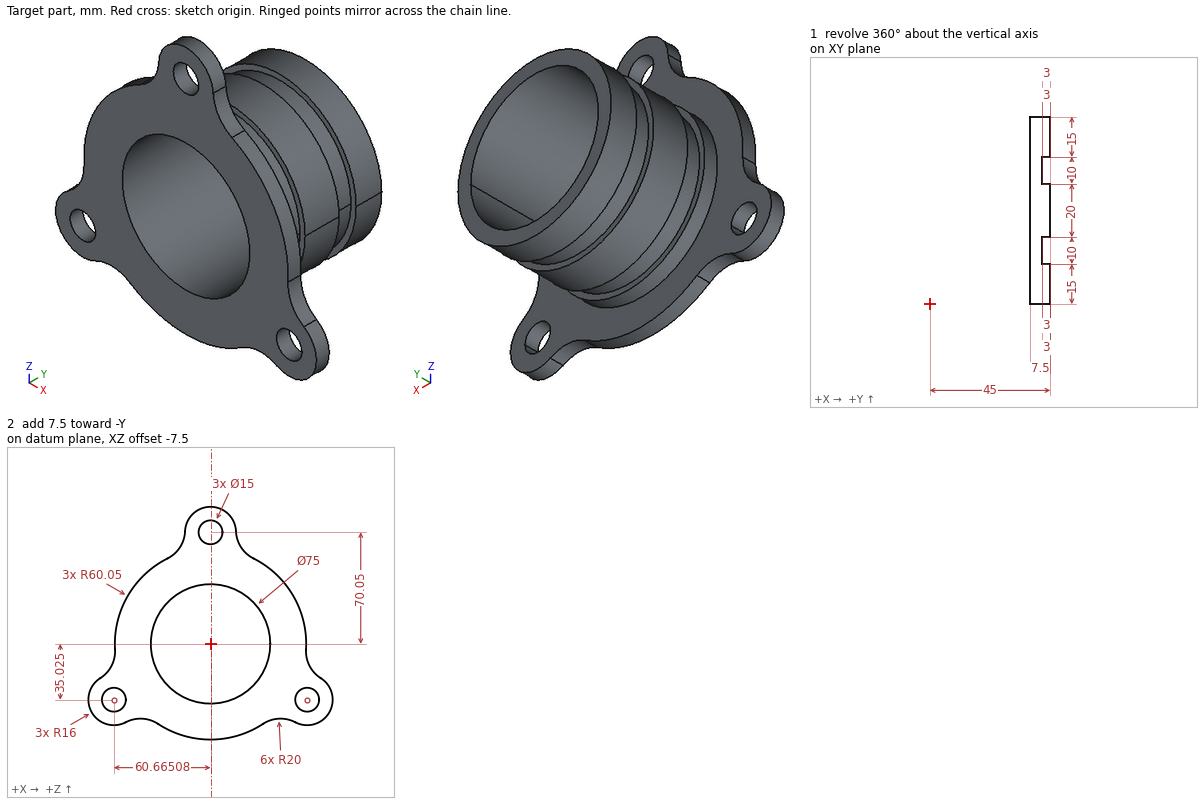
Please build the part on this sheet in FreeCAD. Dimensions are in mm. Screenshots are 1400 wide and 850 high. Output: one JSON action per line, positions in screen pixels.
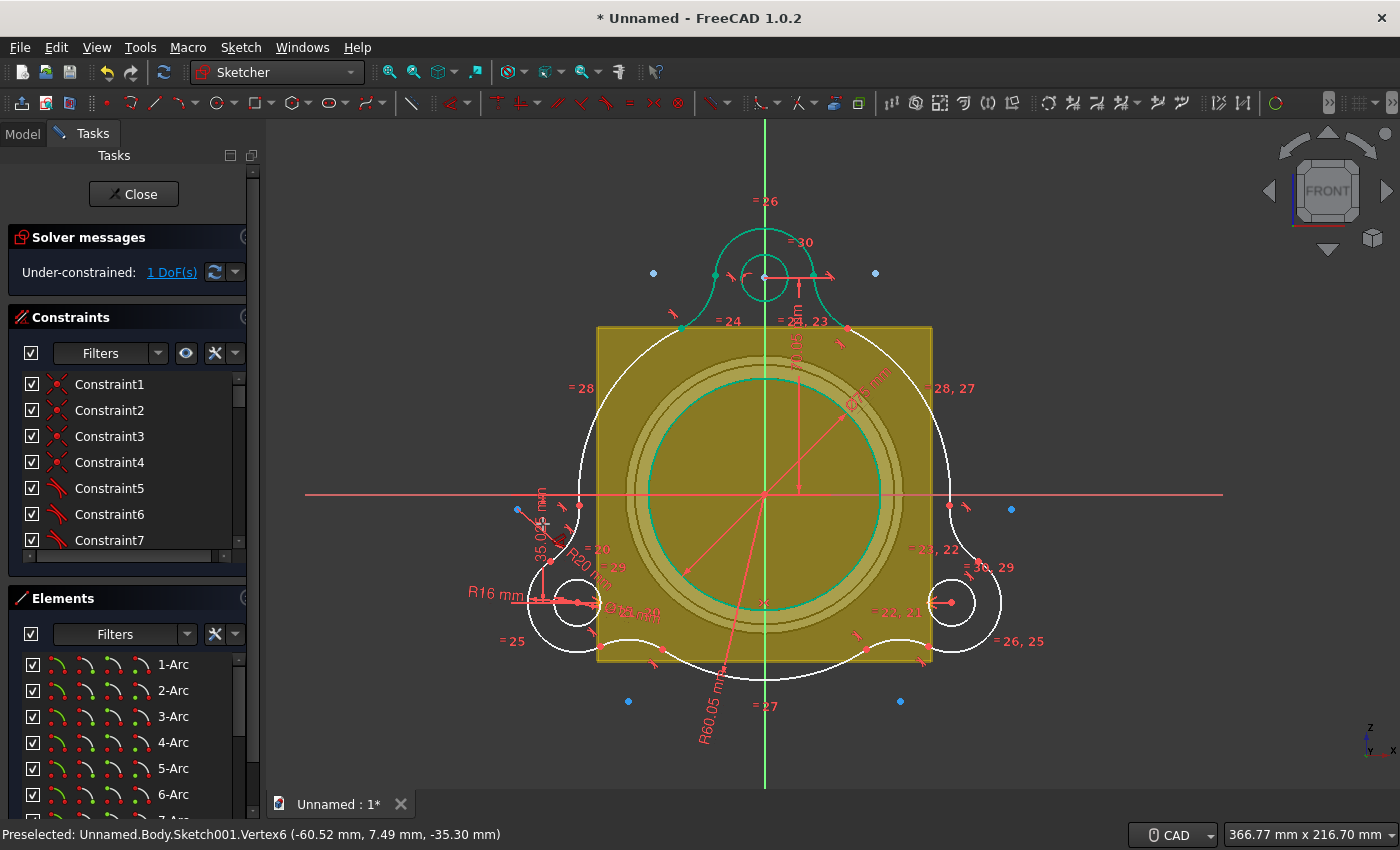
{"action": "left_click", "coordinate": [577, 603]}
{"action": "left_click", "coordinate": [671, 637]}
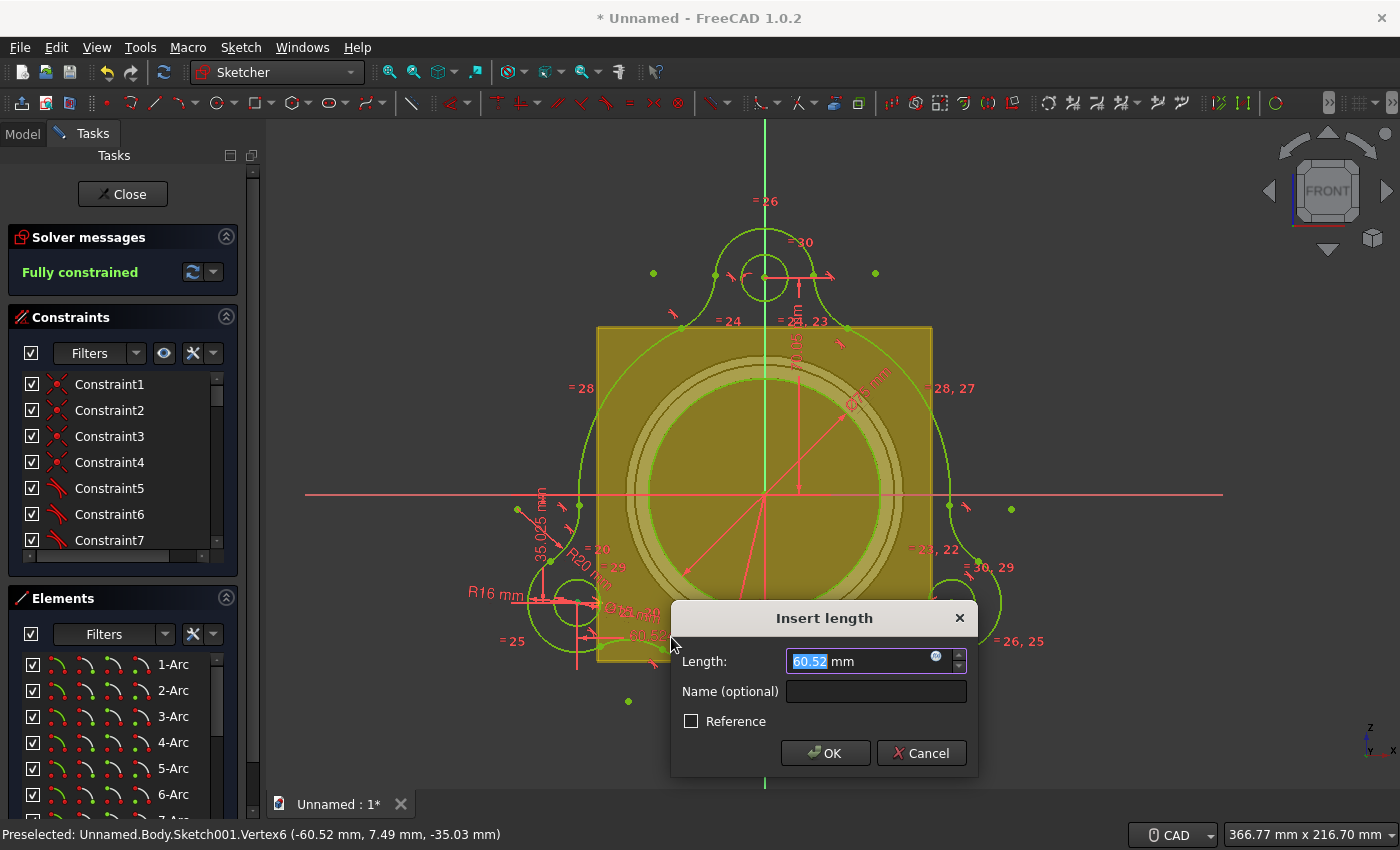
{"action": "type", "text": "60.66508"}
{"action": "key", "text": "Return"}
{"action": "key", "text": "Escape"}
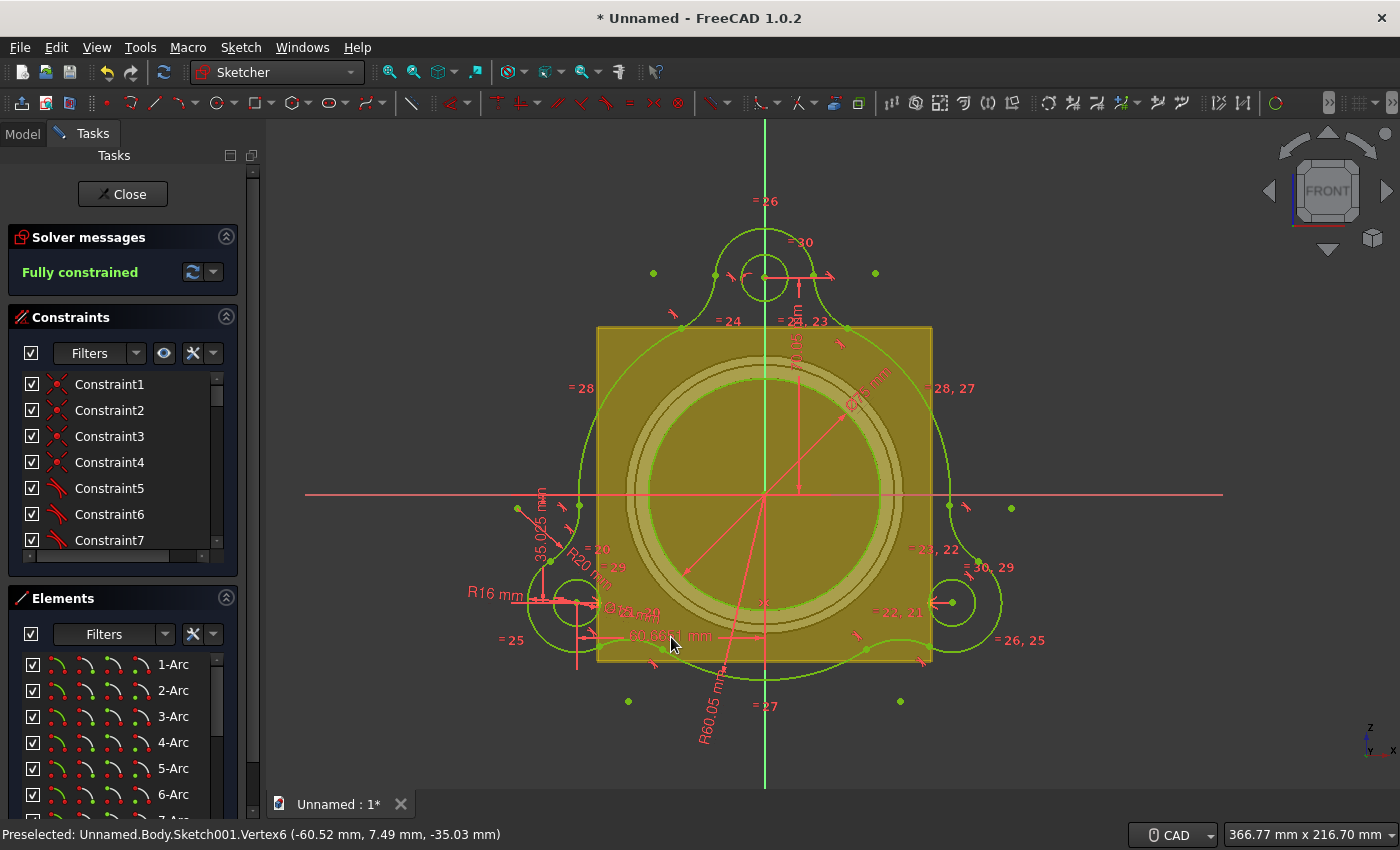
{"action": "left_click", "coordinate": [123, 194]}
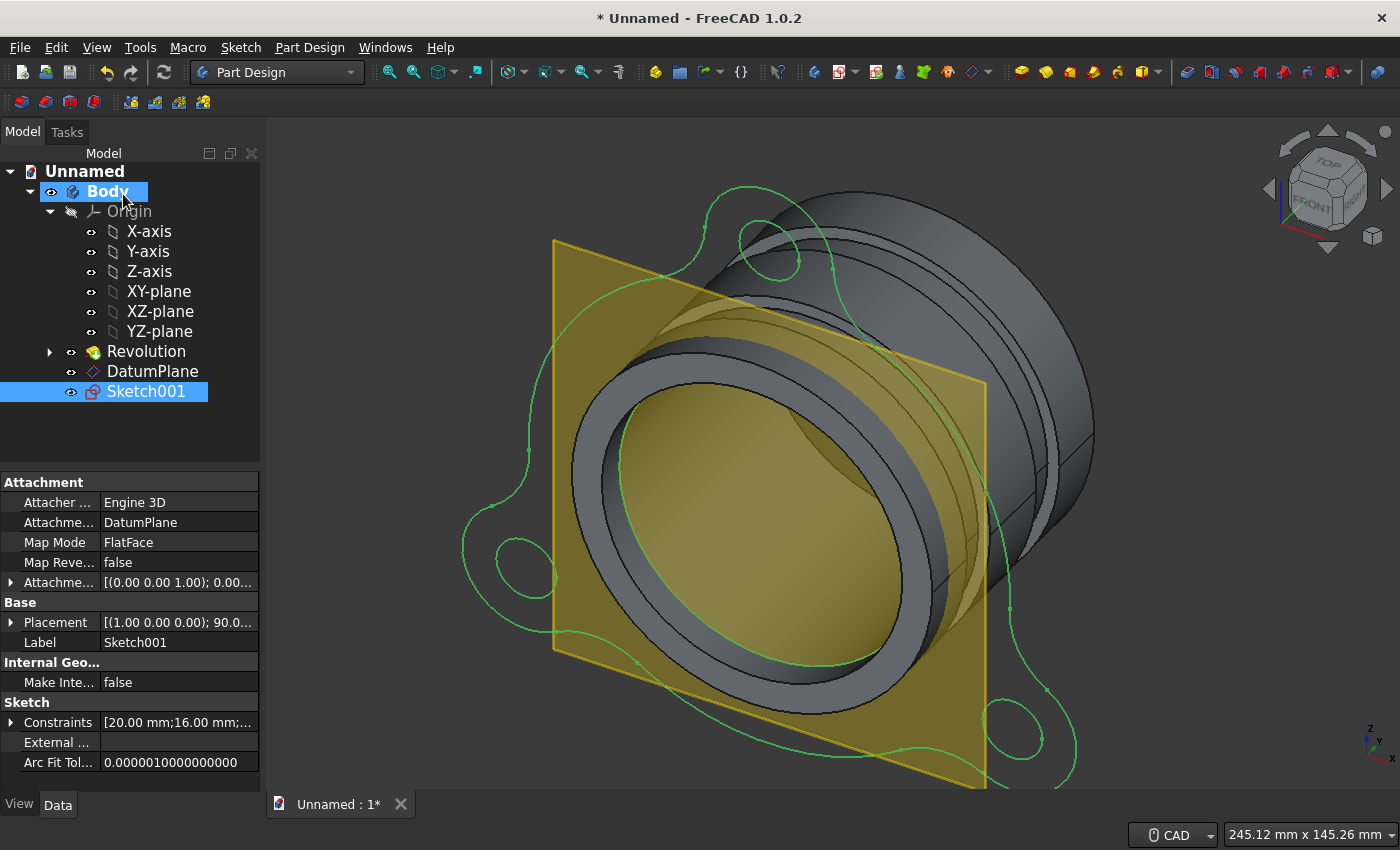
{"action": "left_click", "coordinate": [1022, 72]}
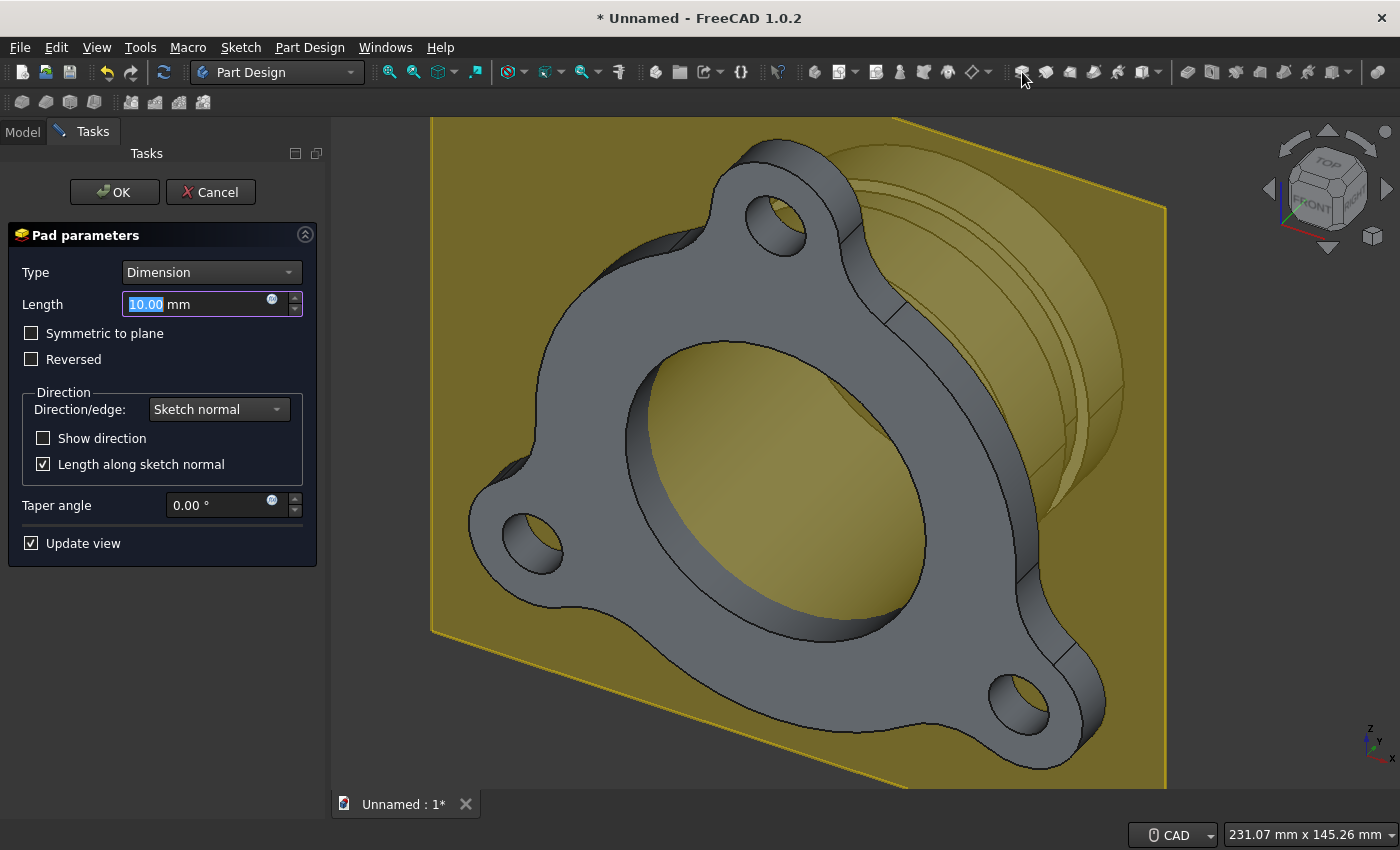
{"action": "type", "text": "7.5"}
{"action": "key", "text": "Tab"}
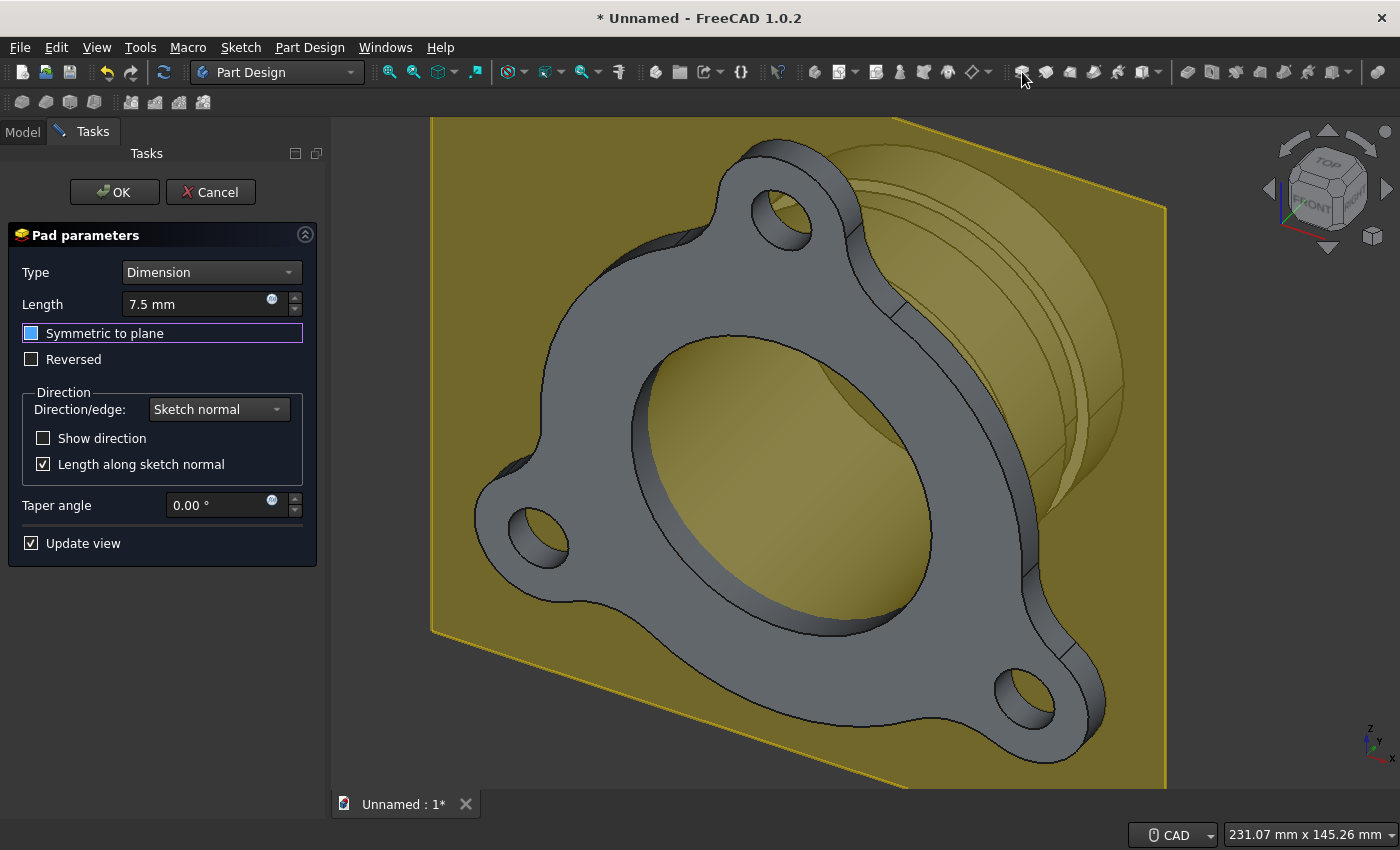
{"action": "left_click", "coordinate": [115, 192]}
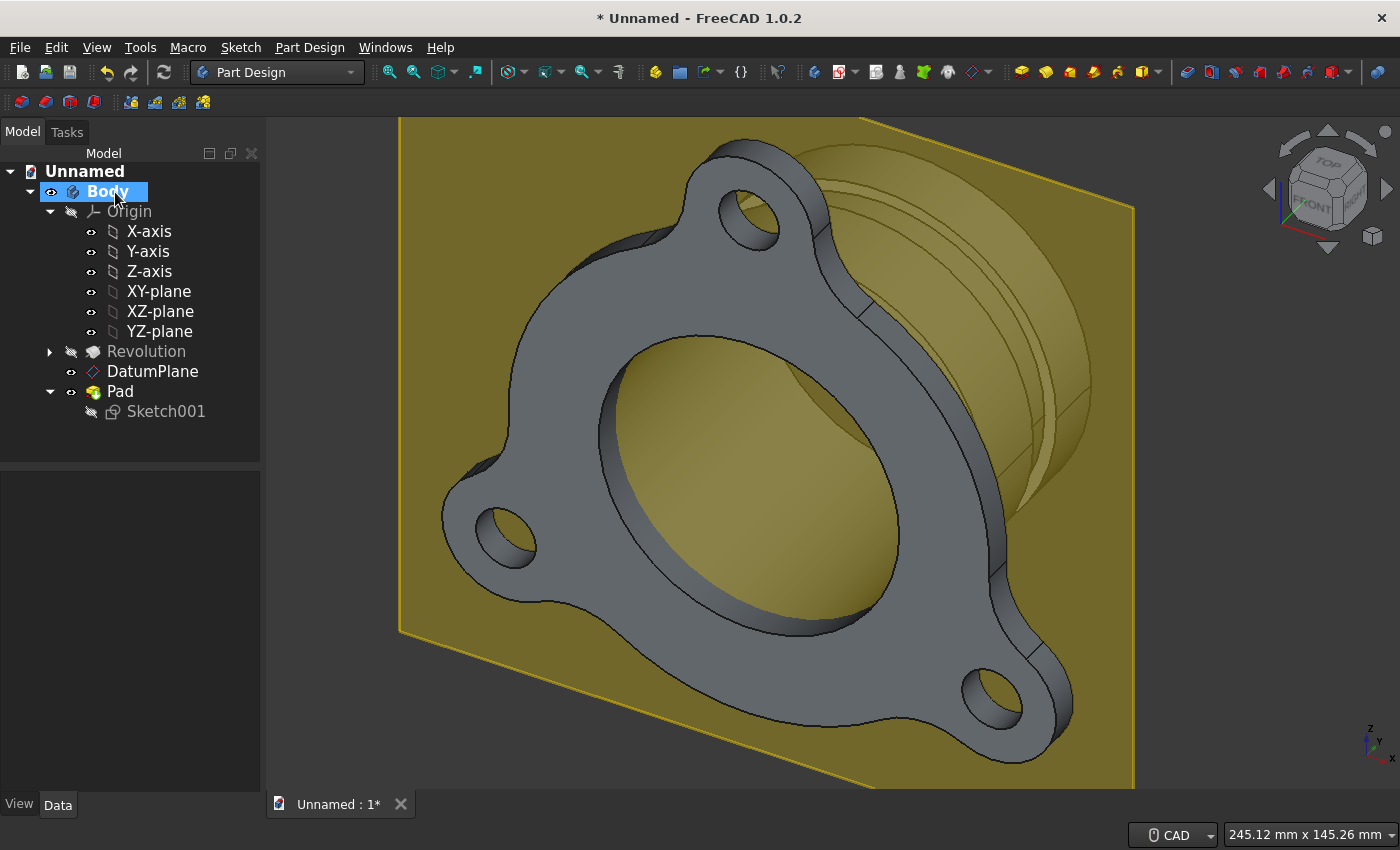
{"action": "left_click", "coordinate": [116, 372]}
{"action": "key", "text": "space"}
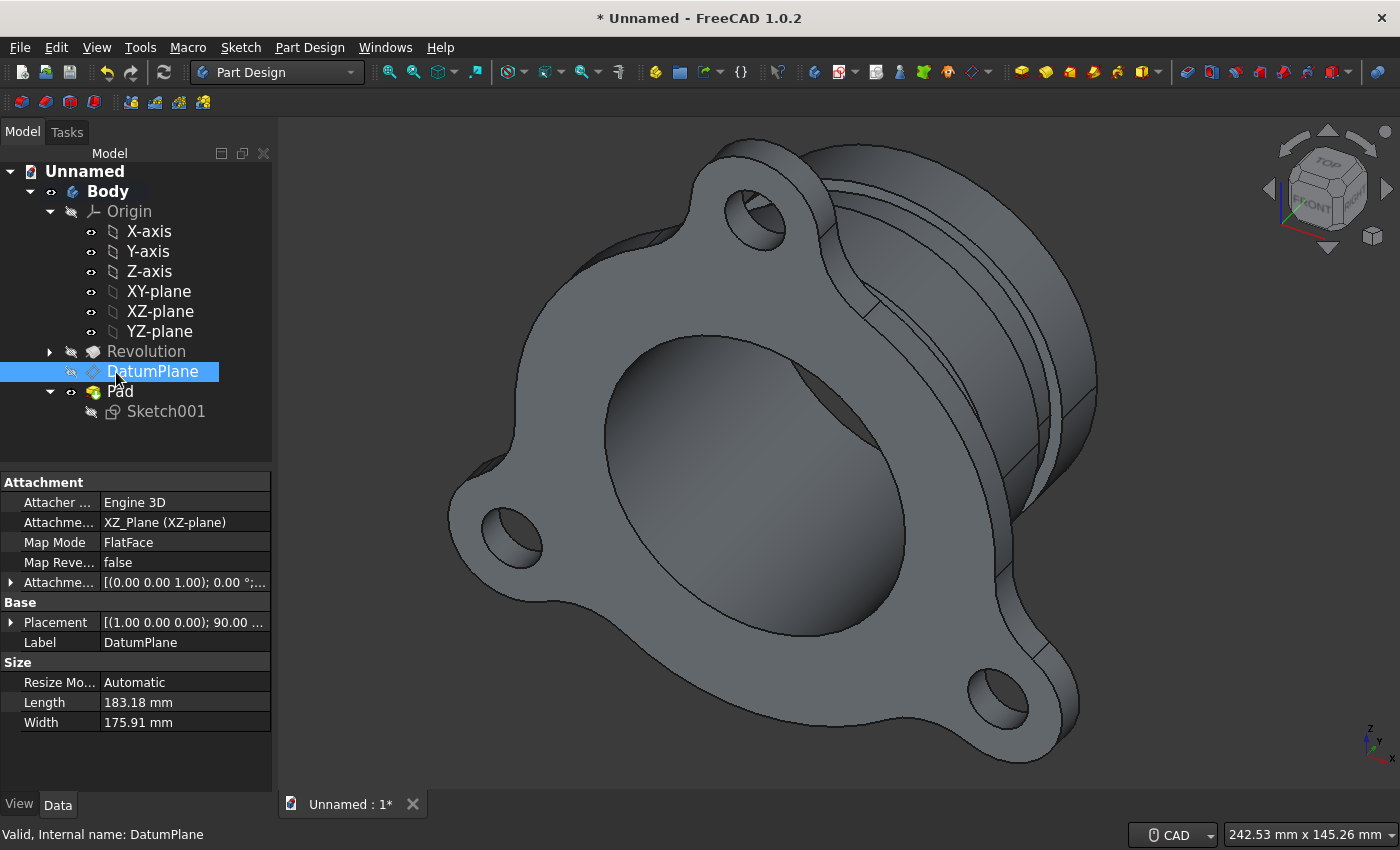
{"action": "key", "text": "0"}